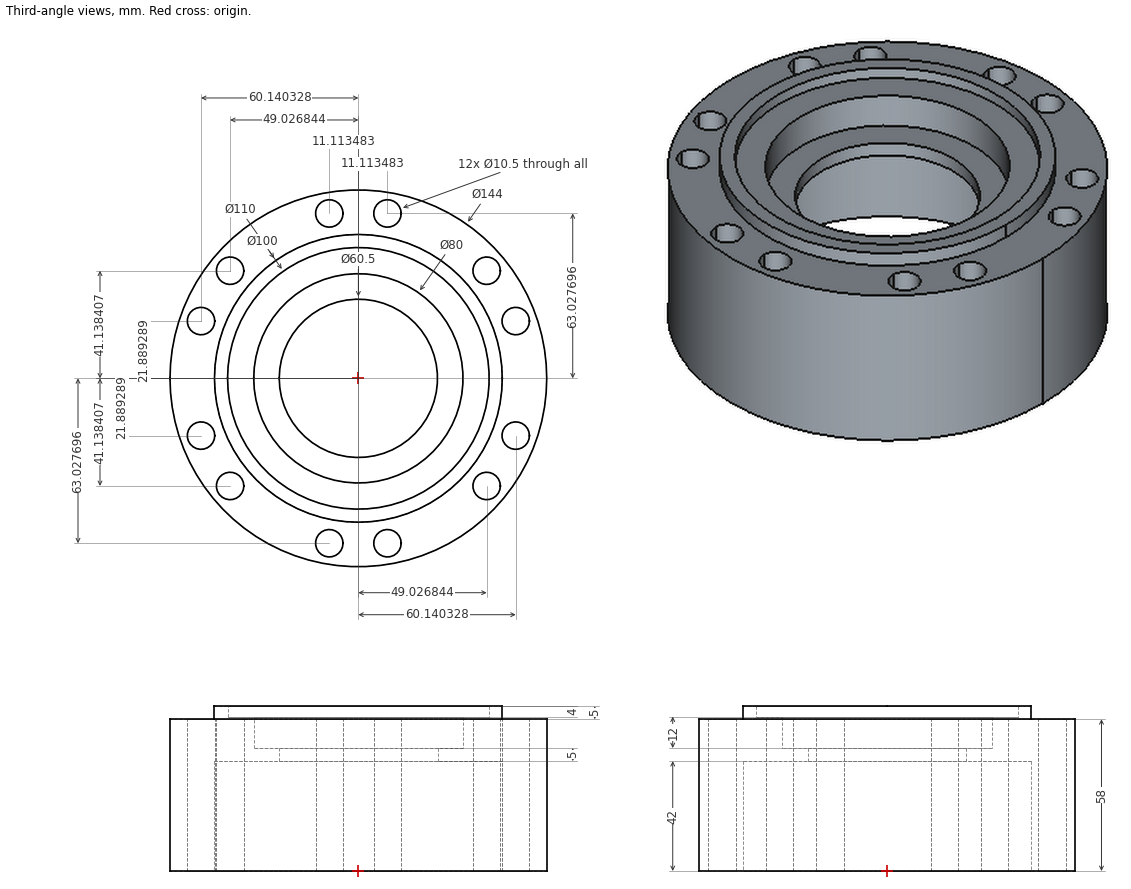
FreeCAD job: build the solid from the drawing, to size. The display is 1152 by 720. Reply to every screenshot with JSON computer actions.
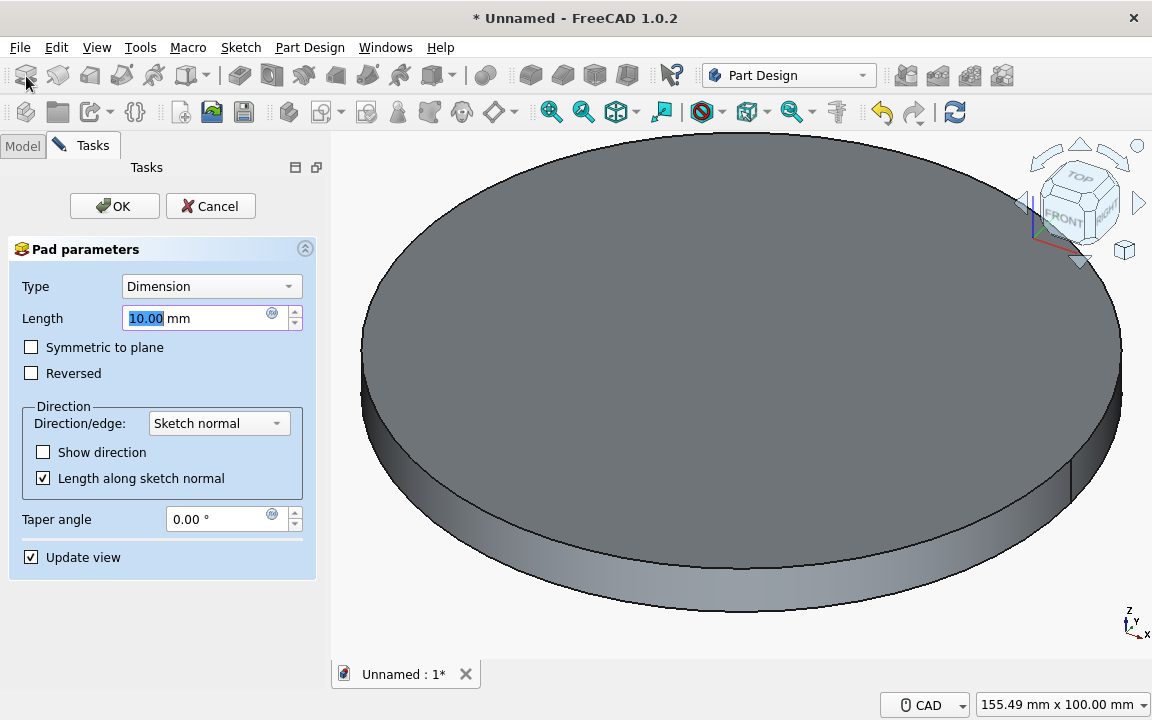
{"action": "type", "text": "58"}
{"action": "key", "text": "Tab"}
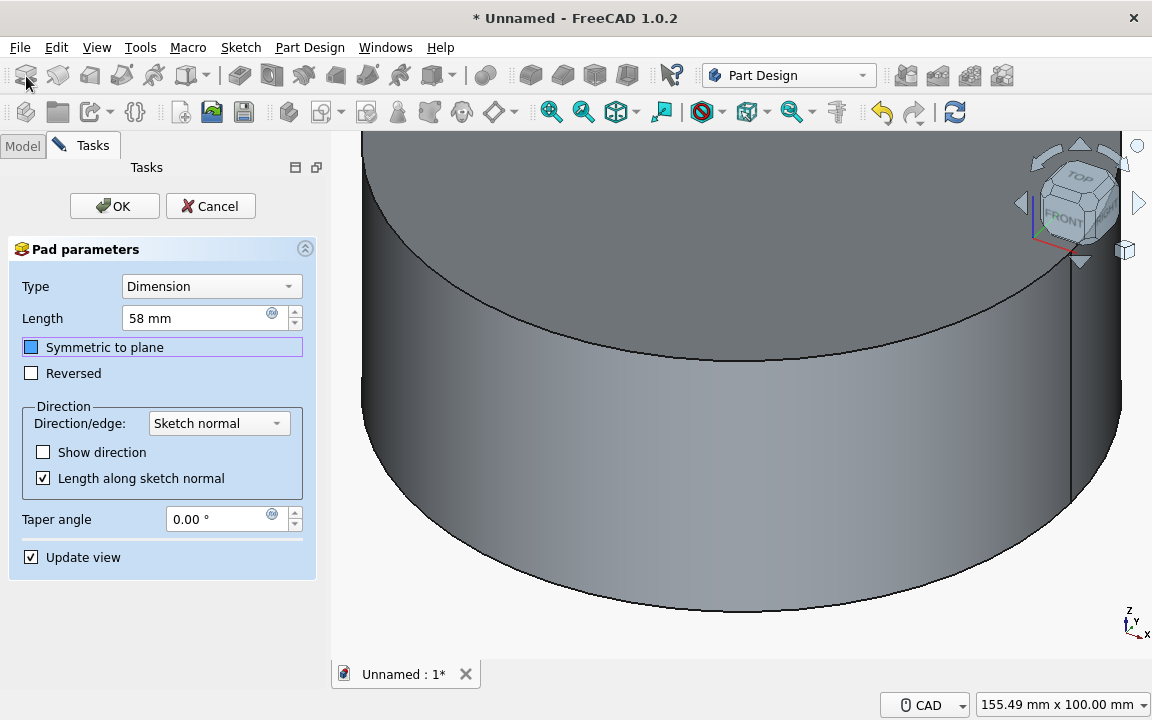
{"action": "left_click", "coordinate": [115, 206]}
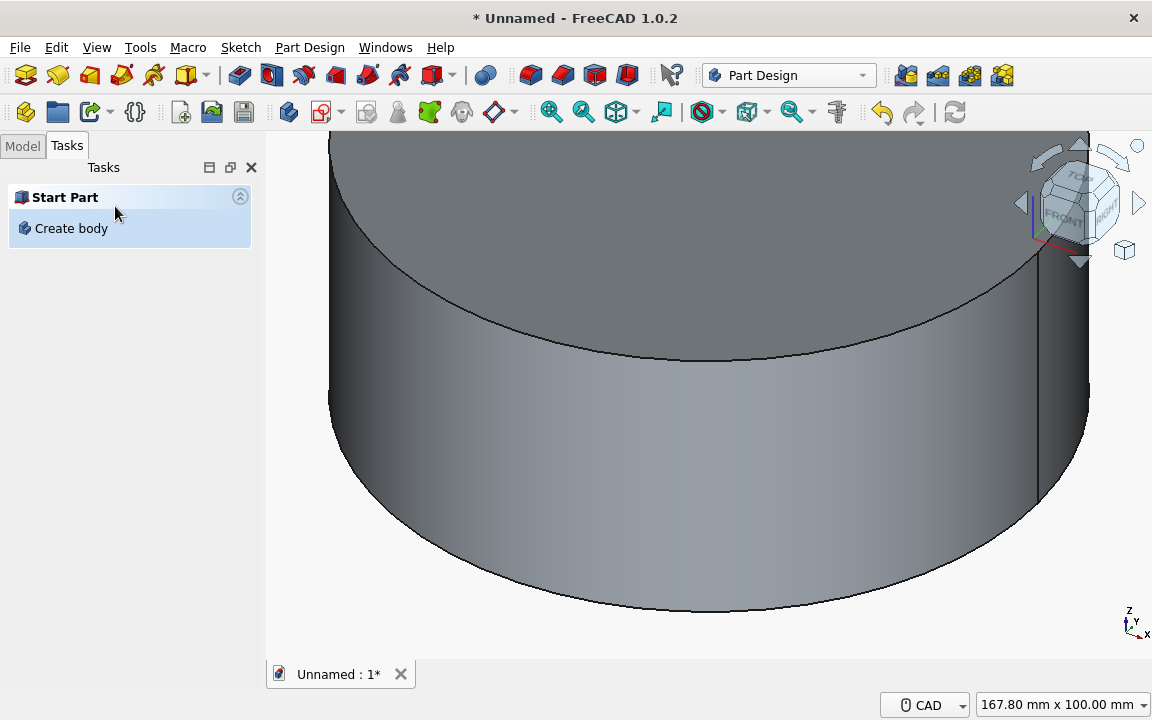
{"action": "key", "text": "v f"}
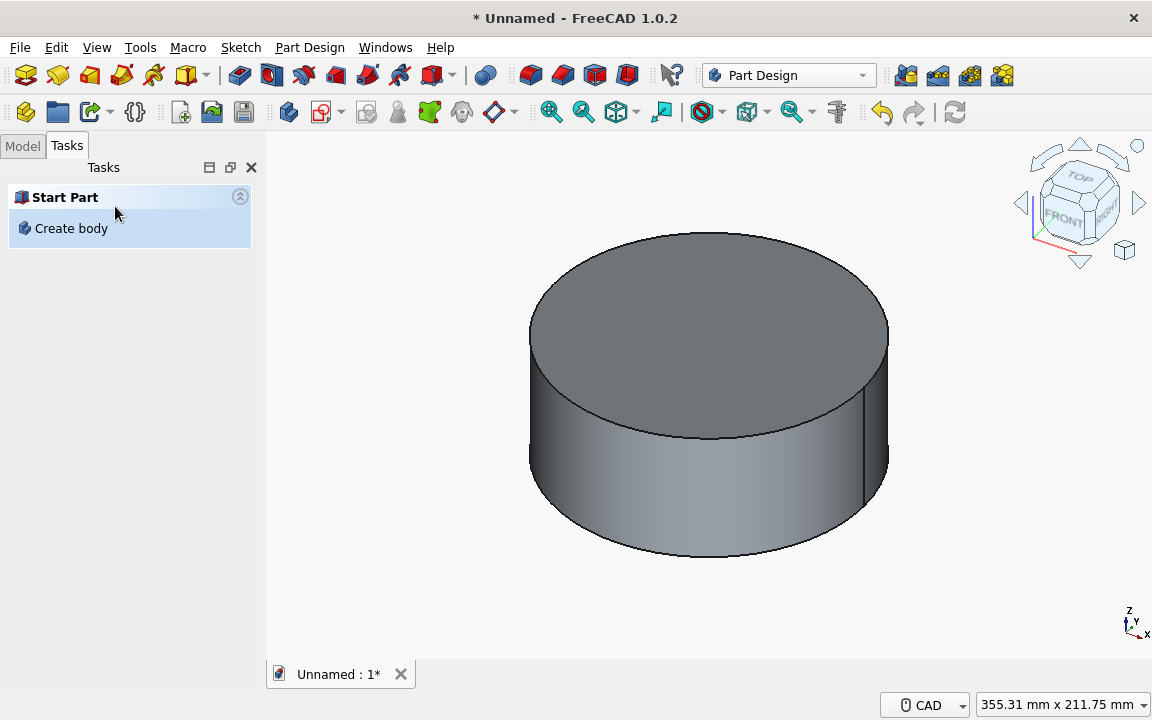
{"action": "left_click", "coordinate": [709, 335]}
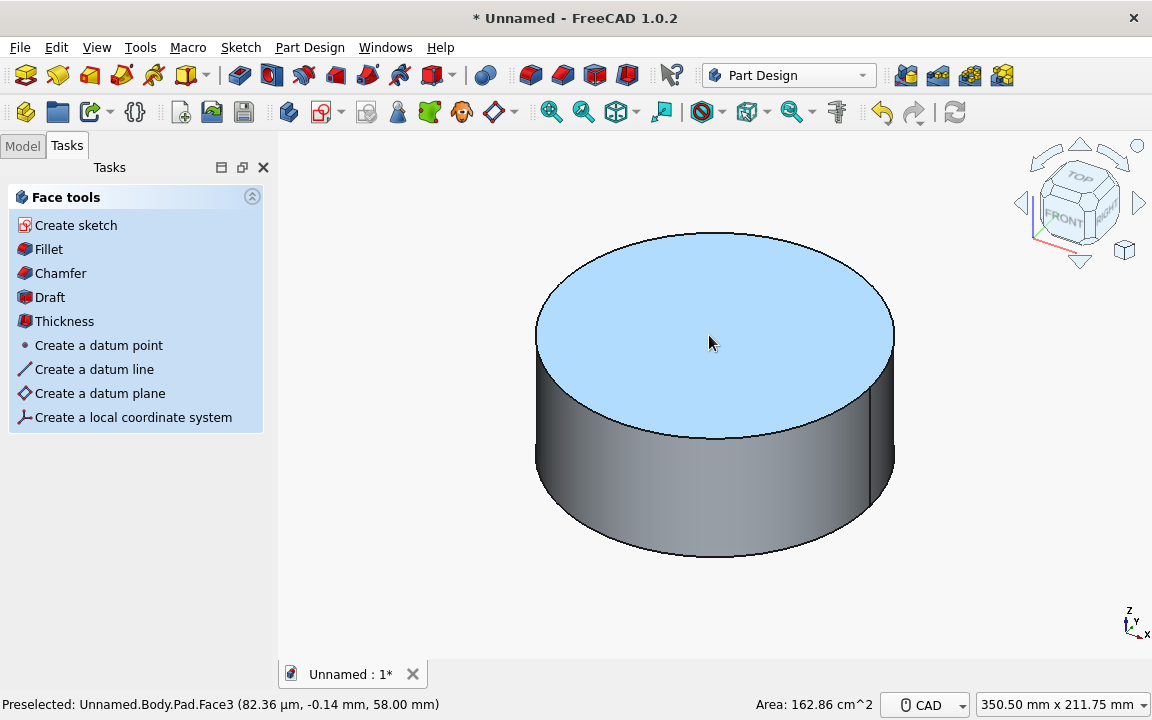
{"action": "left_click", "coordinate": [322, 112]}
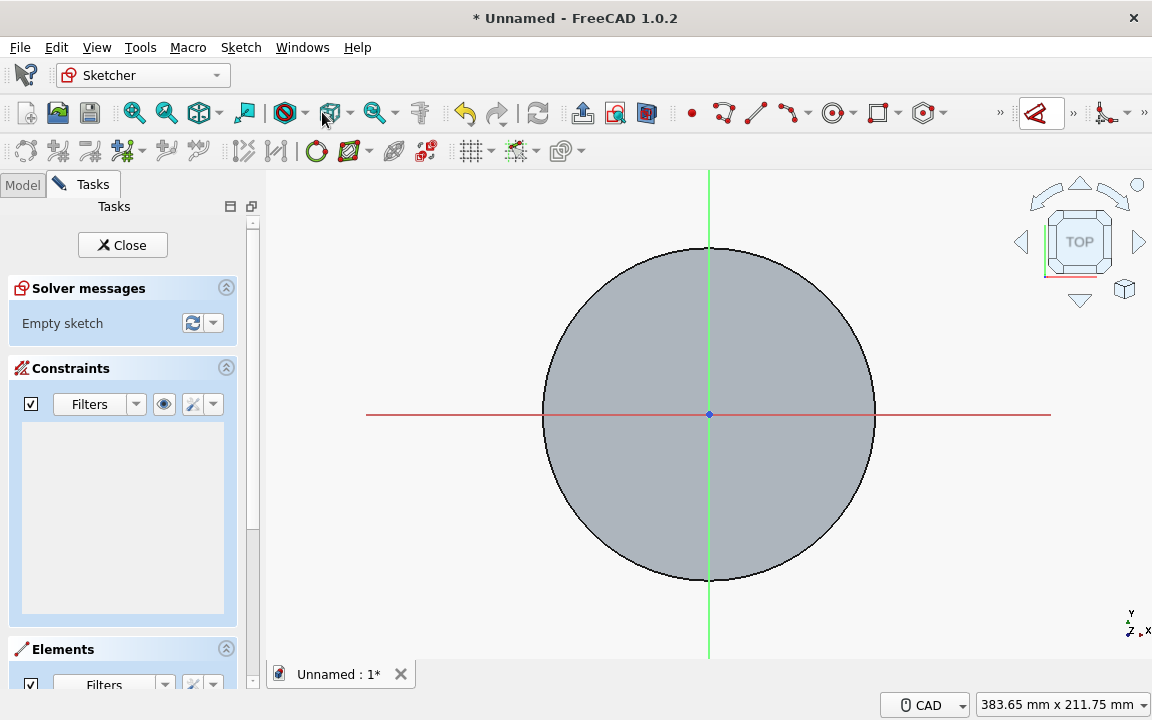
{"action": "key", "text": "g c"}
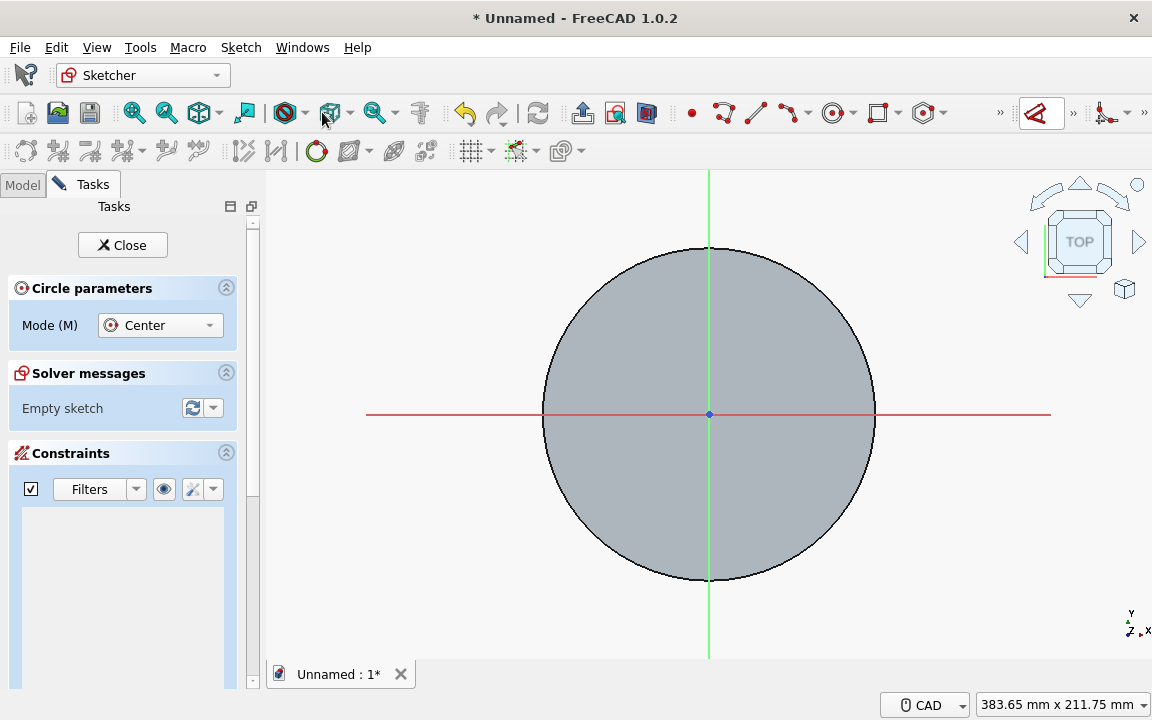
{"action": "left_click", "coordinate": [709, 414]}
{"action": "left_click", "coordinate": [799, 325]}
{"action": "key", "text": "Escape"}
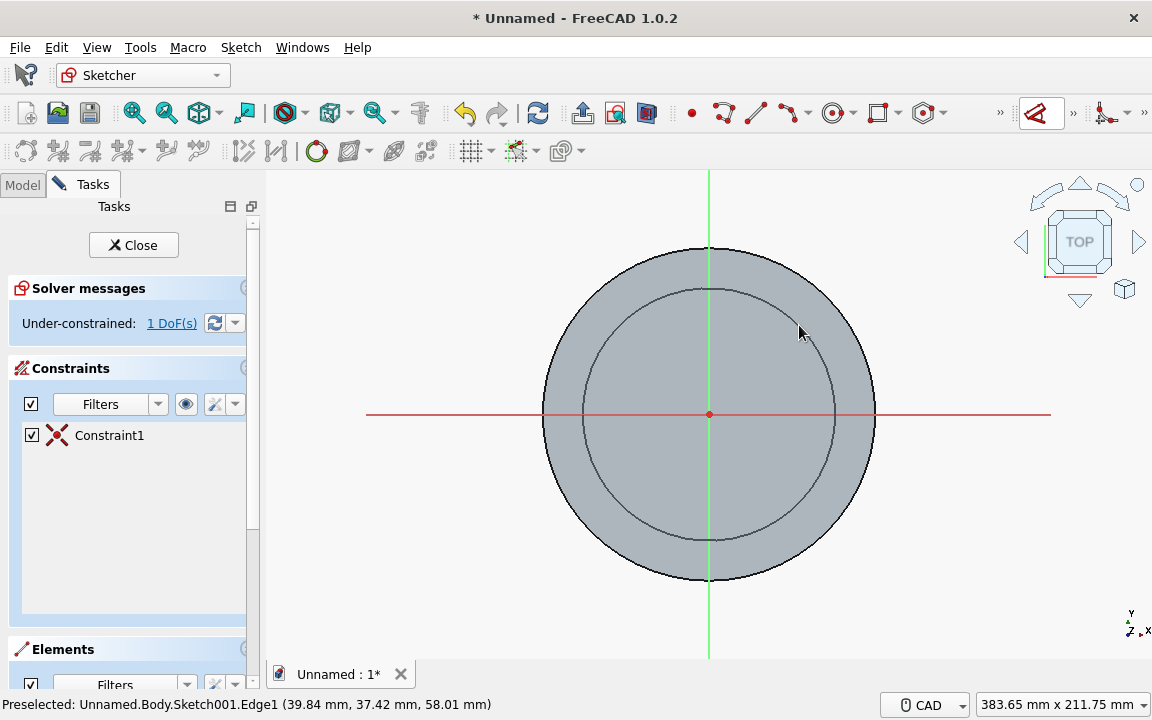
{"action": "key", "text": "d"}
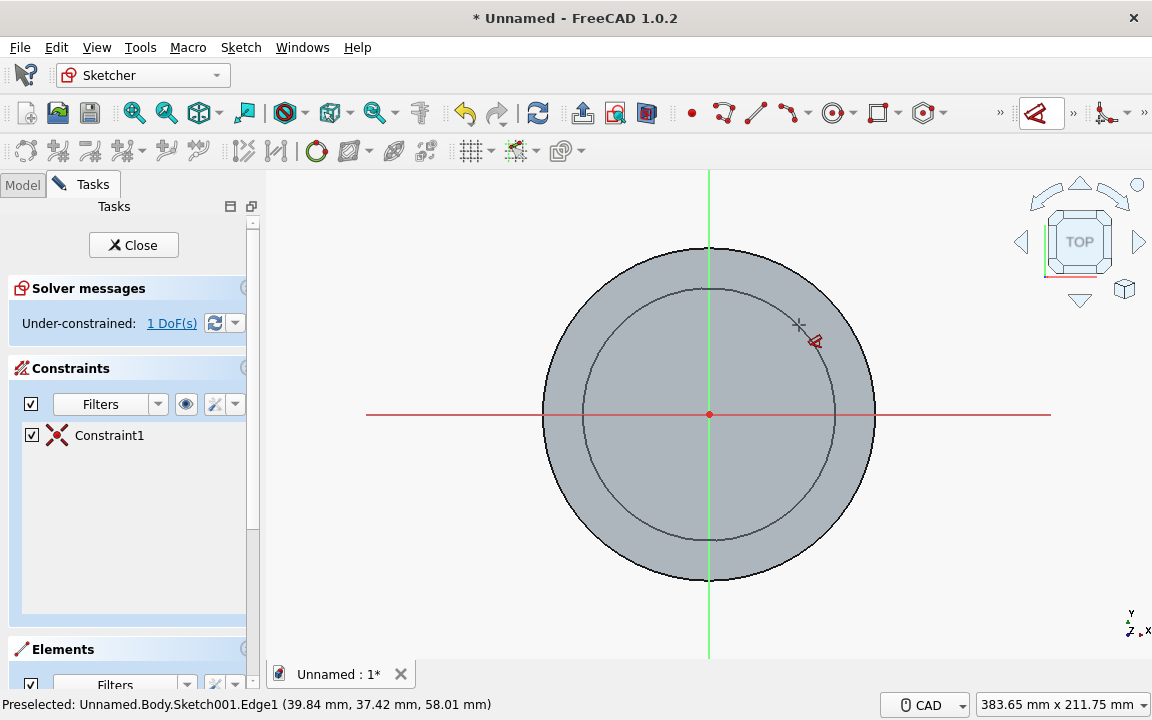
{"action": "left_click", "coordinate": [798, 325]}
{"action": "left_click", "coordinate": [821, 302]}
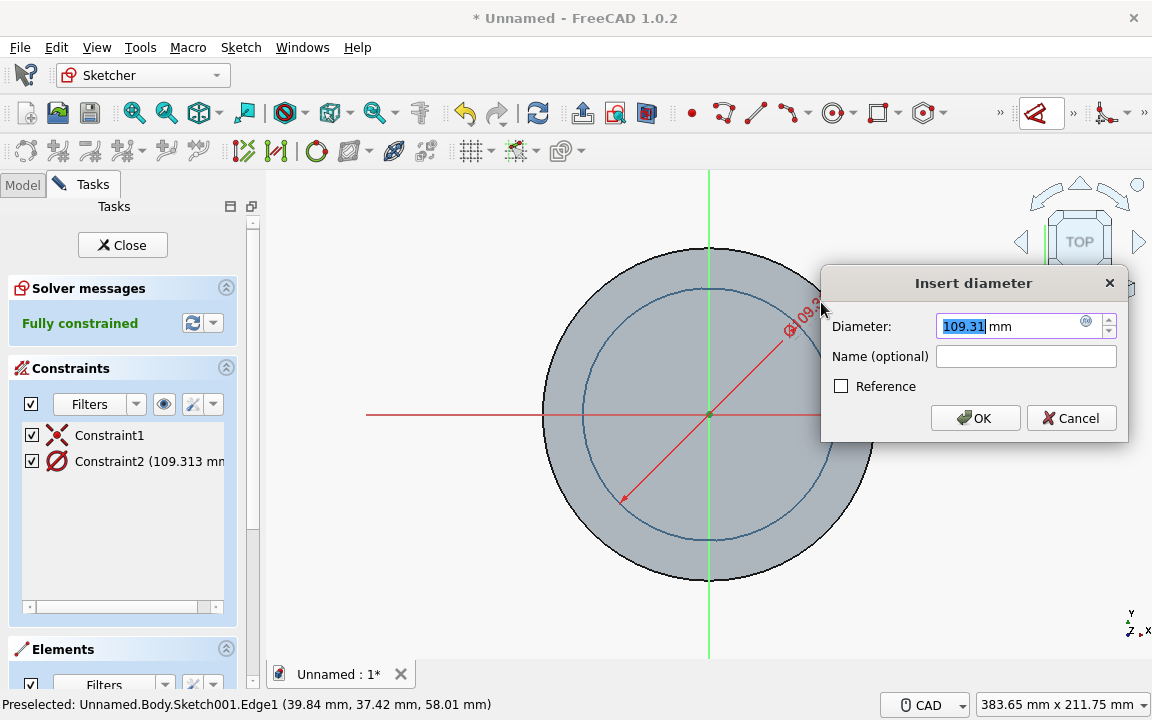
{"action": "type", "text": "110"}
{"action": "key", "text": "Return"}
{"action": "key", "text": "Escape"}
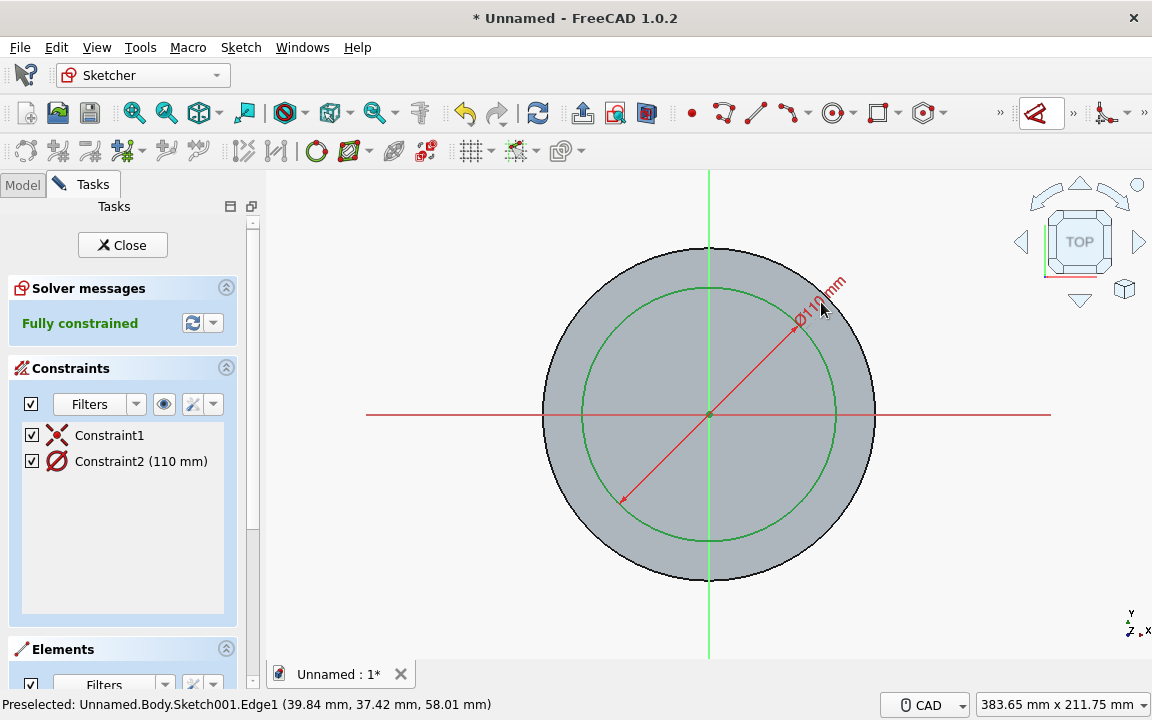
{"action": "left_click", "coordinate": [123, 245]}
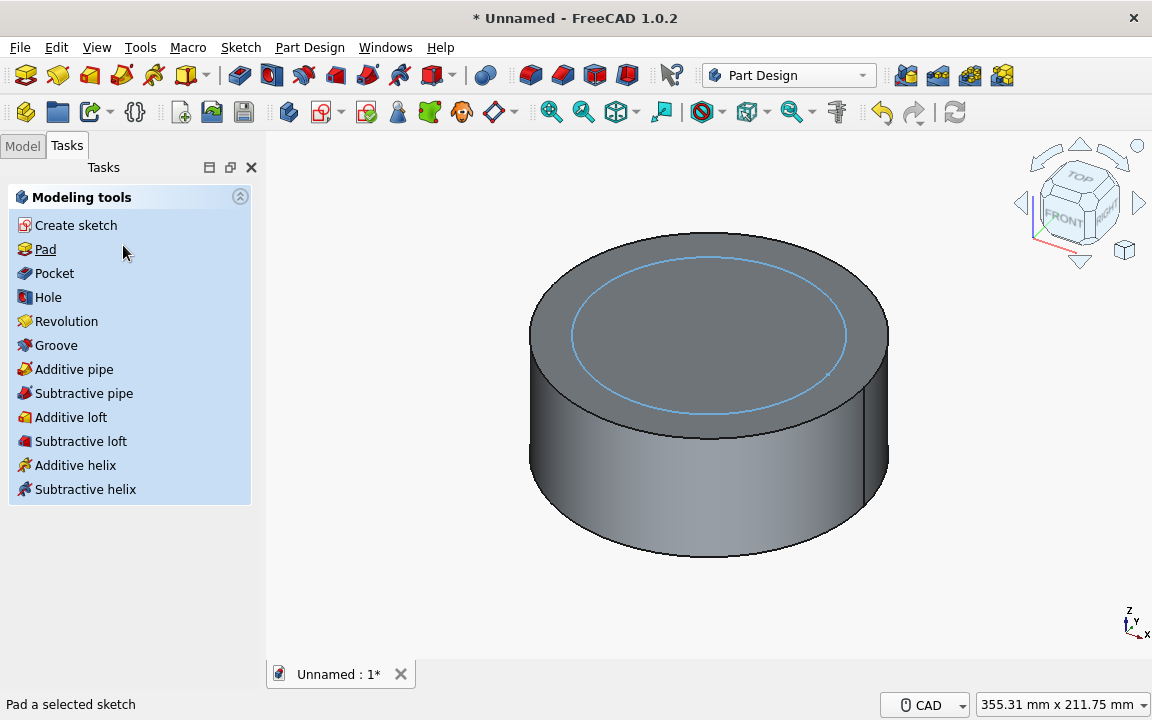
{"action": "left_click", "coordinate": [26, 76]}